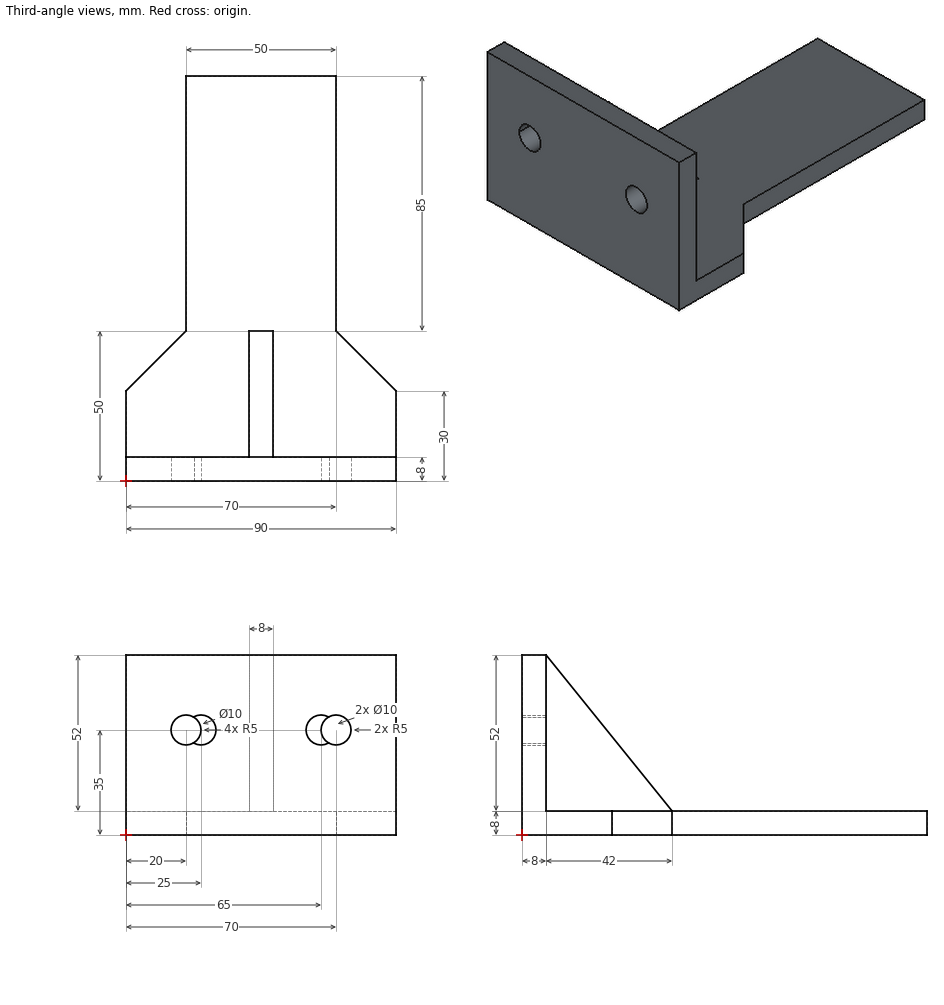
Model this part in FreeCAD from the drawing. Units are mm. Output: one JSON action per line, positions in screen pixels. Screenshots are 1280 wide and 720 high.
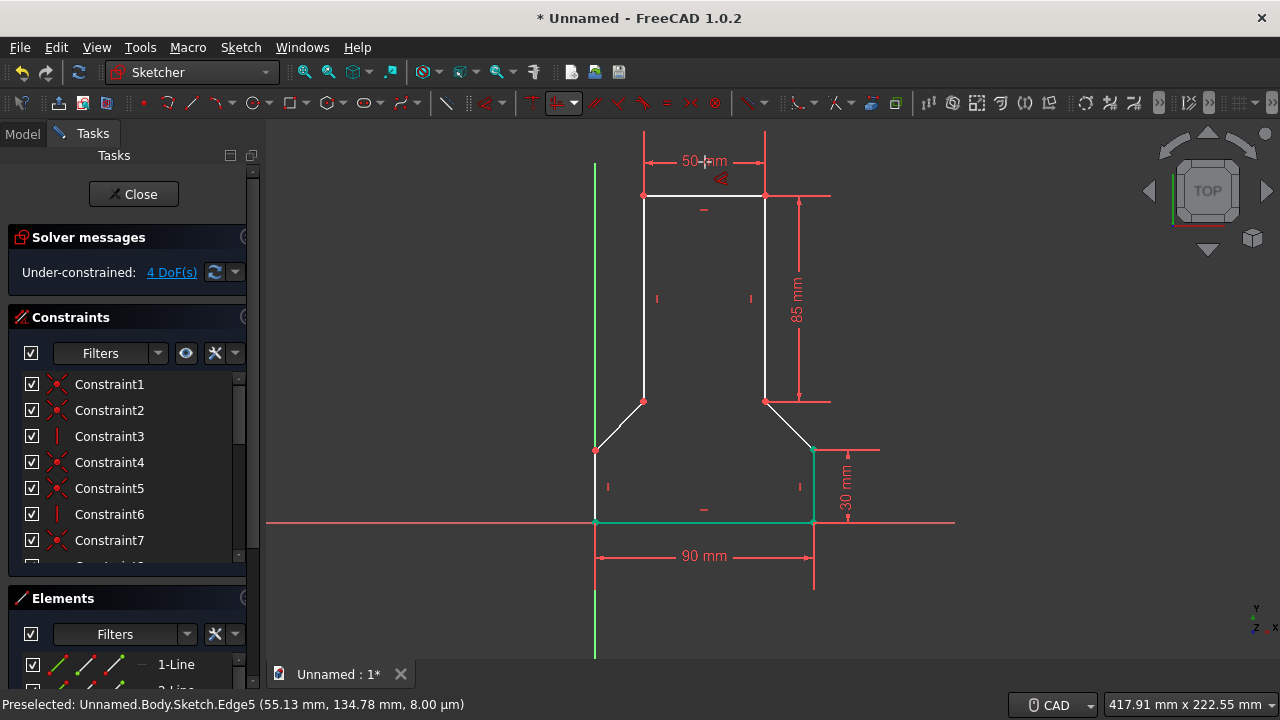
{"action": "left_click", "coordinate": [644, 258]}
{"action": "left_click", "coordinate": [610, 299]}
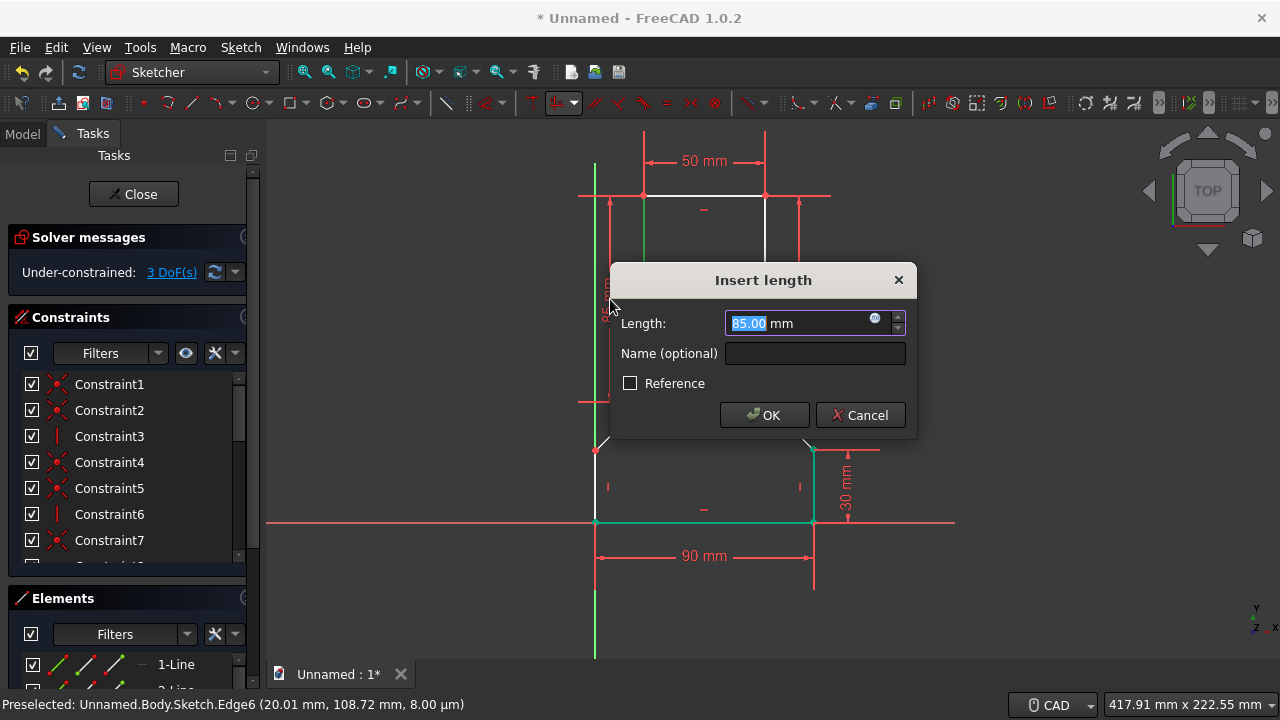
{"action": "type", "text": "85"}
{"action": "key", "text": "Return"}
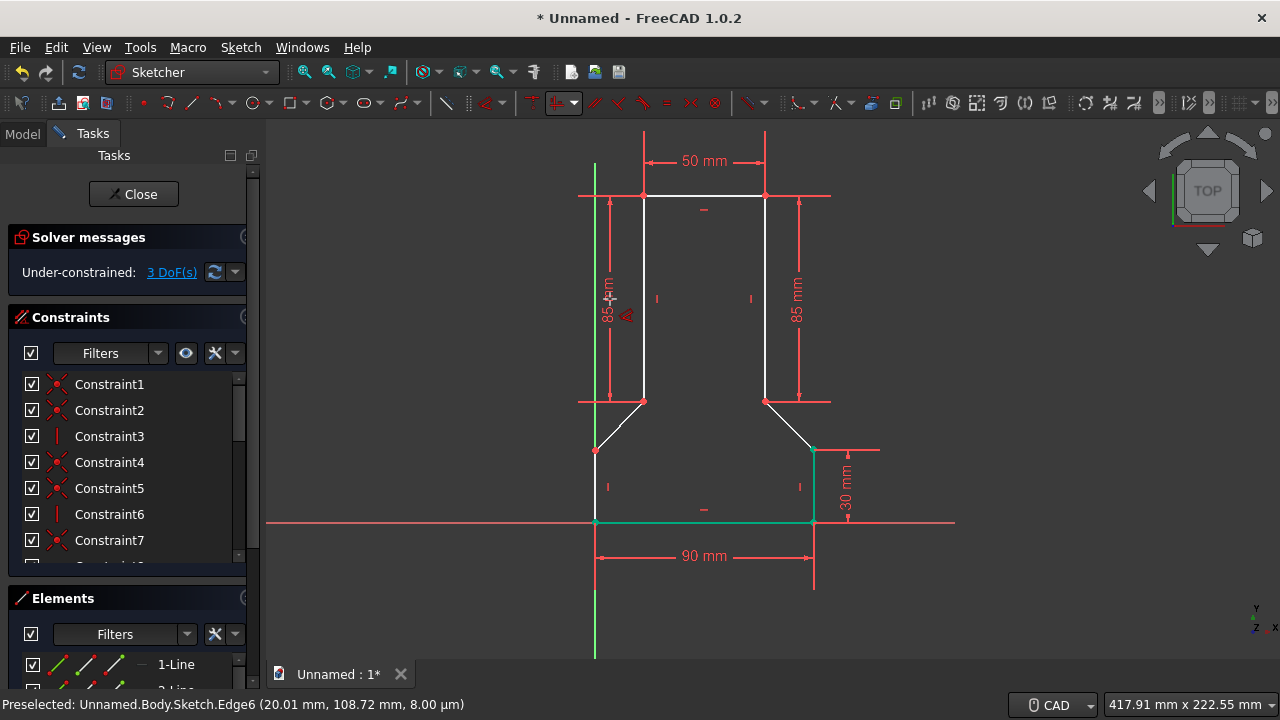
{"action": "left_click", "coordinate": [595, 473]}
{"action": "left_click", "coordinate": [561, 487]}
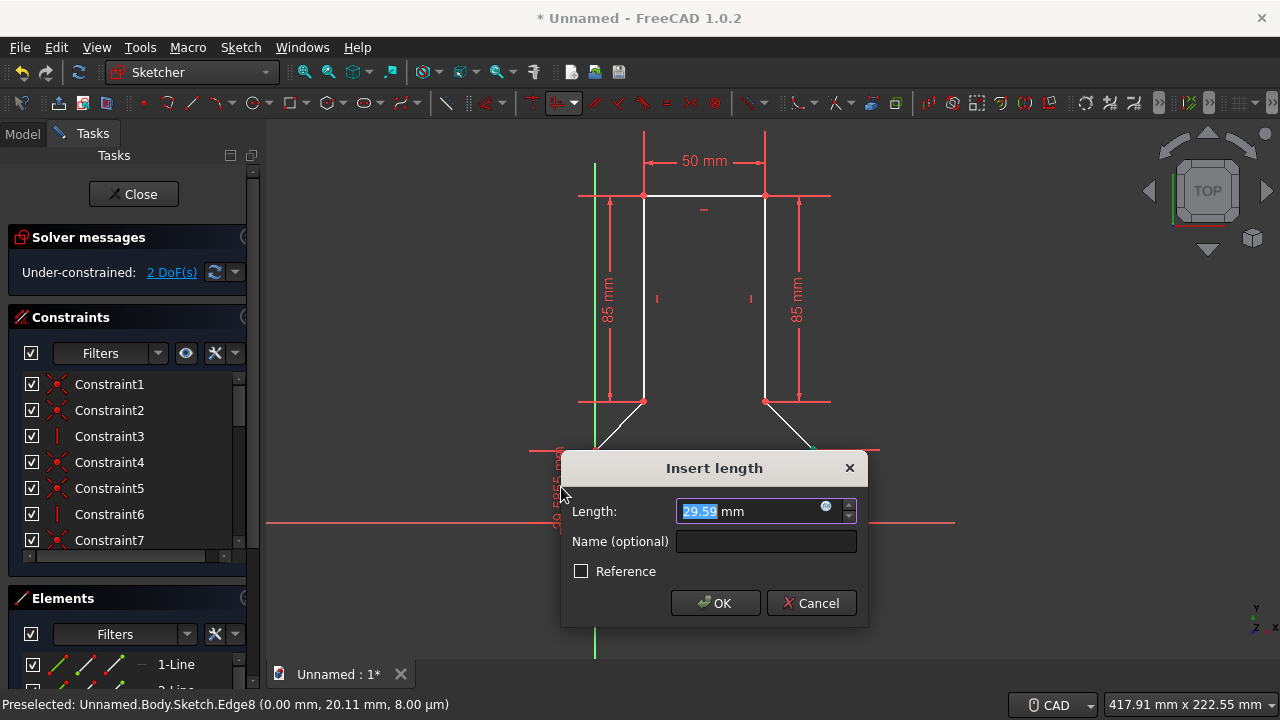
{"action": "type", "text": "30"}
{"action": "key", "text": "Return"}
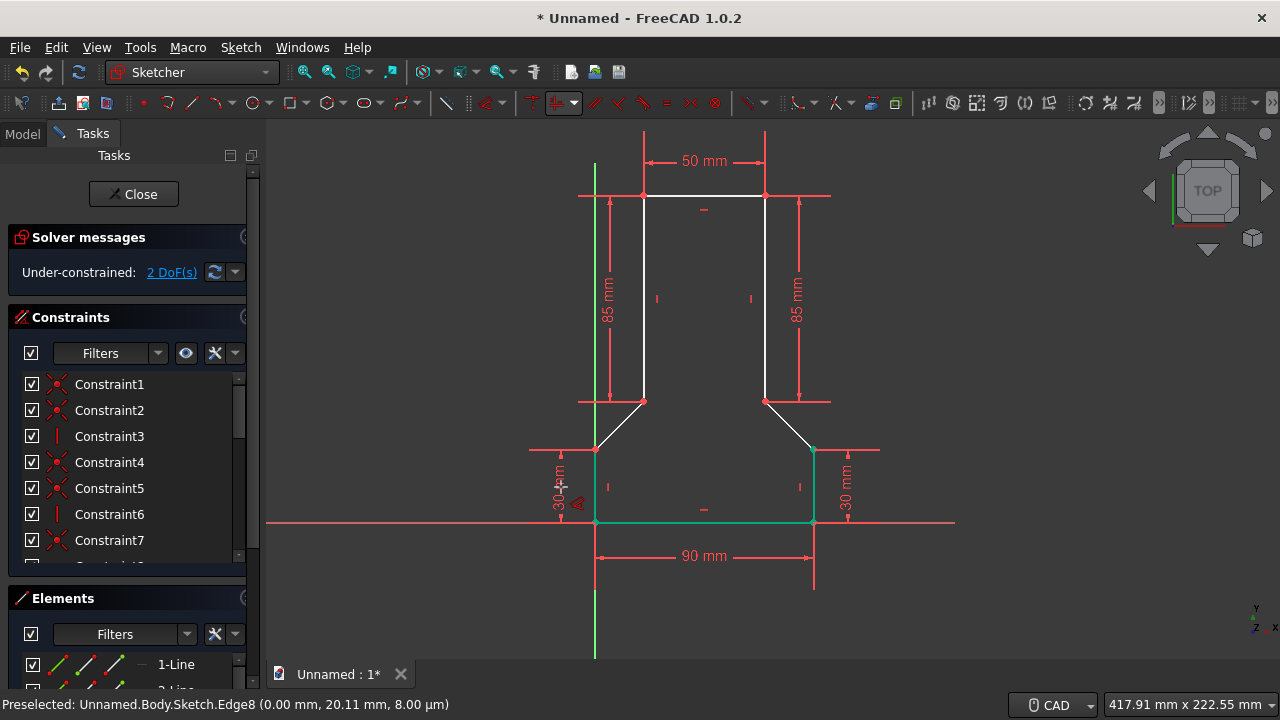
{"action": "left_click", "coordinate": [765, 402]}
{"action": "left_click", "coordinate": [621, 557]}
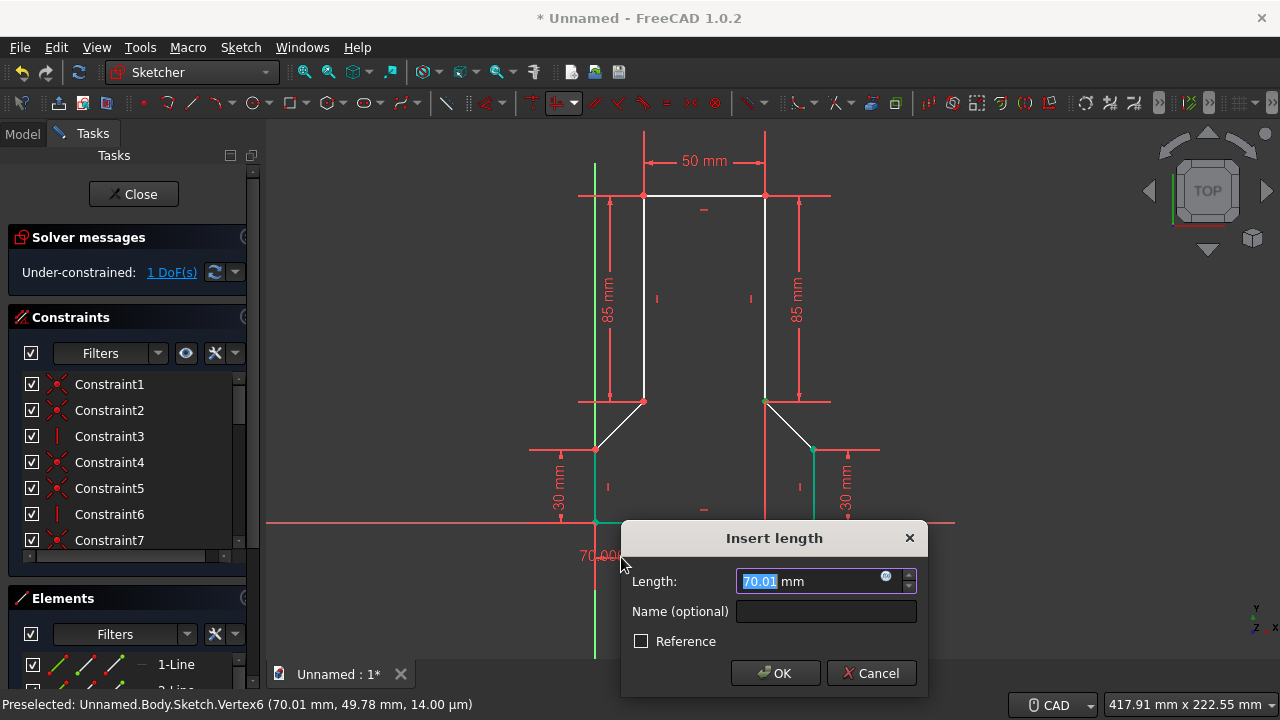
{"action": "type", "text": "70"}
{"action": "key", "text": "Return"}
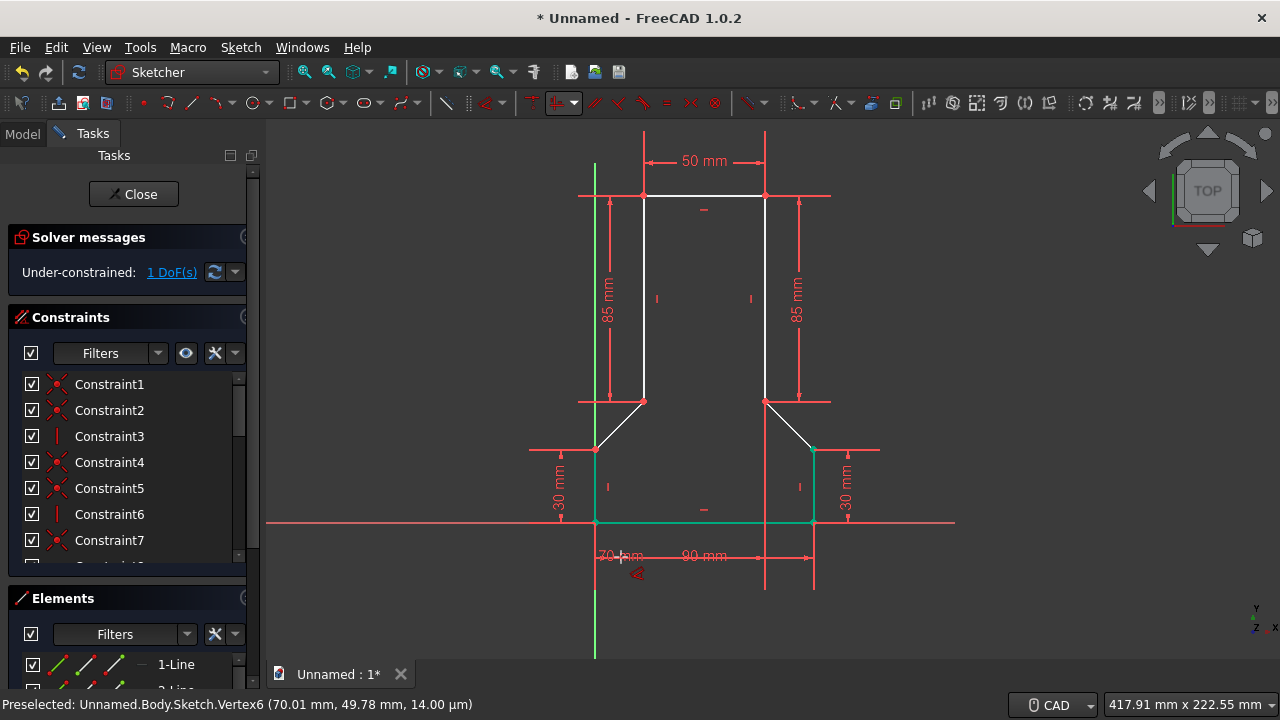
{"action": "left_click", "coordinate": [765, 402]}
{"action": "left_click", "coordinate": [561, 462]}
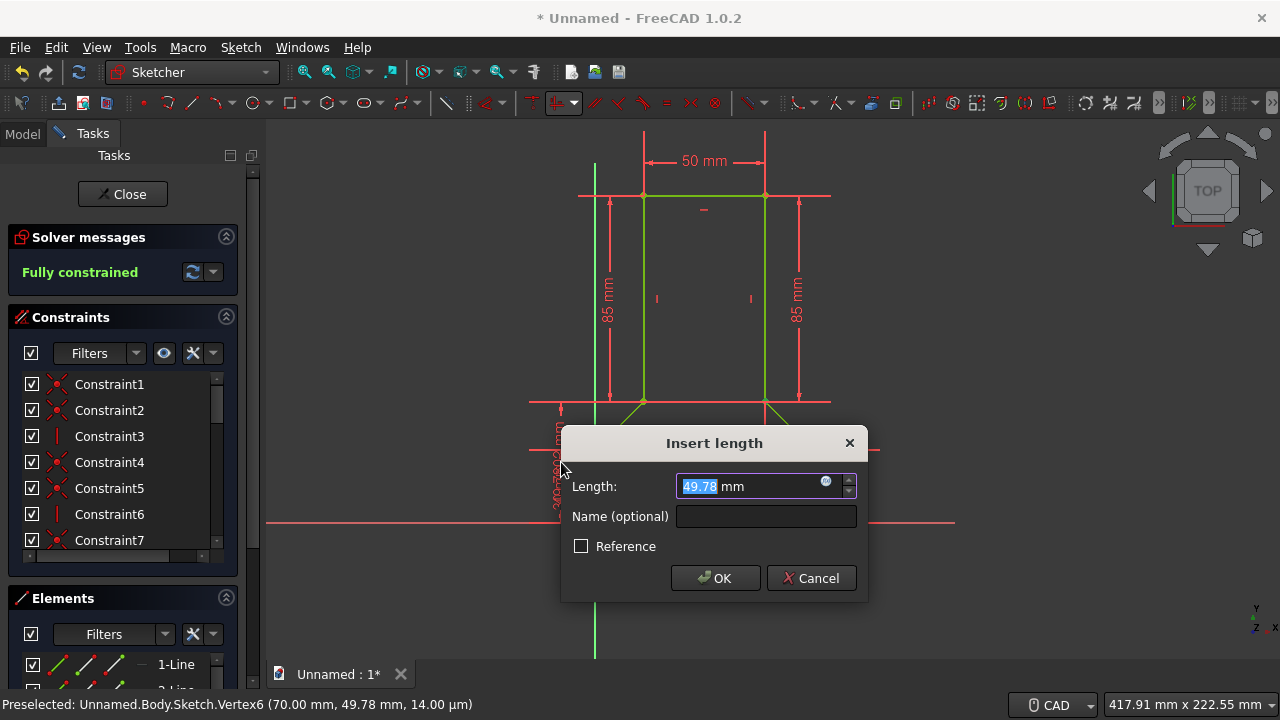
{"action": "type", "text": "50"}
{"action": "key", "text": "Return"}
{"action": "key", "text": "Escape"}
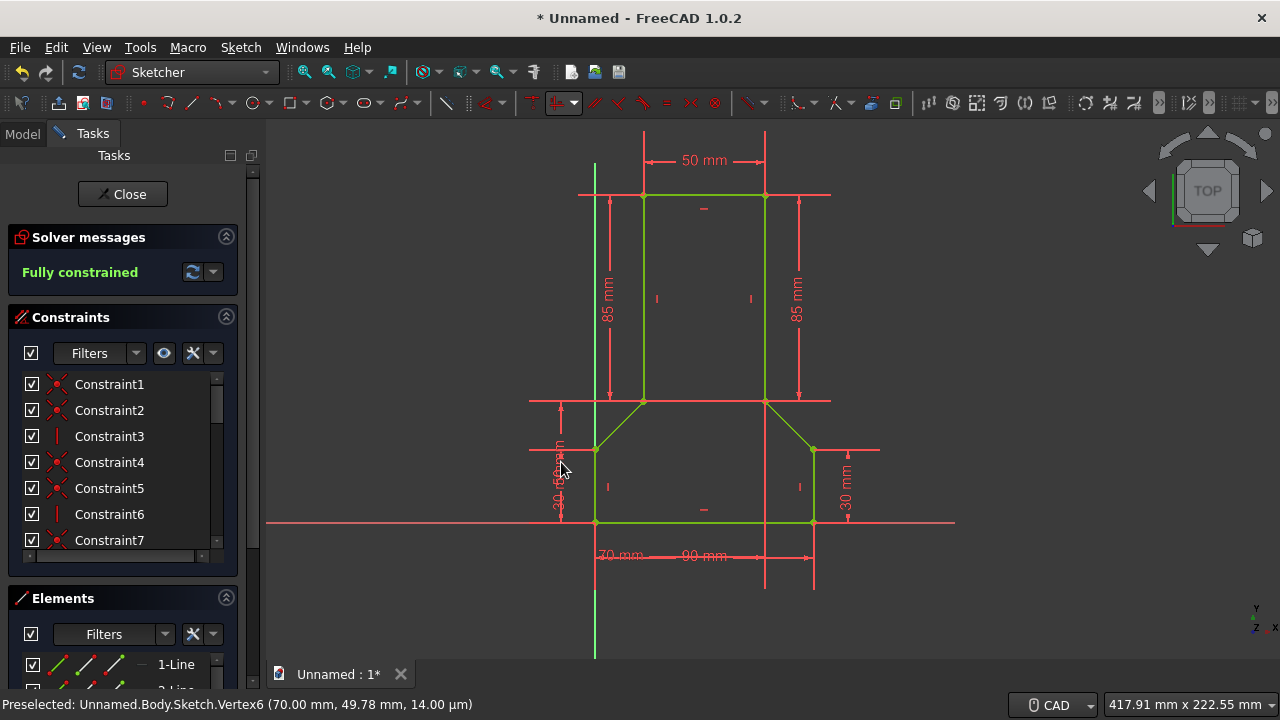
{"action": "left_click", "coordinate": [123, 194]}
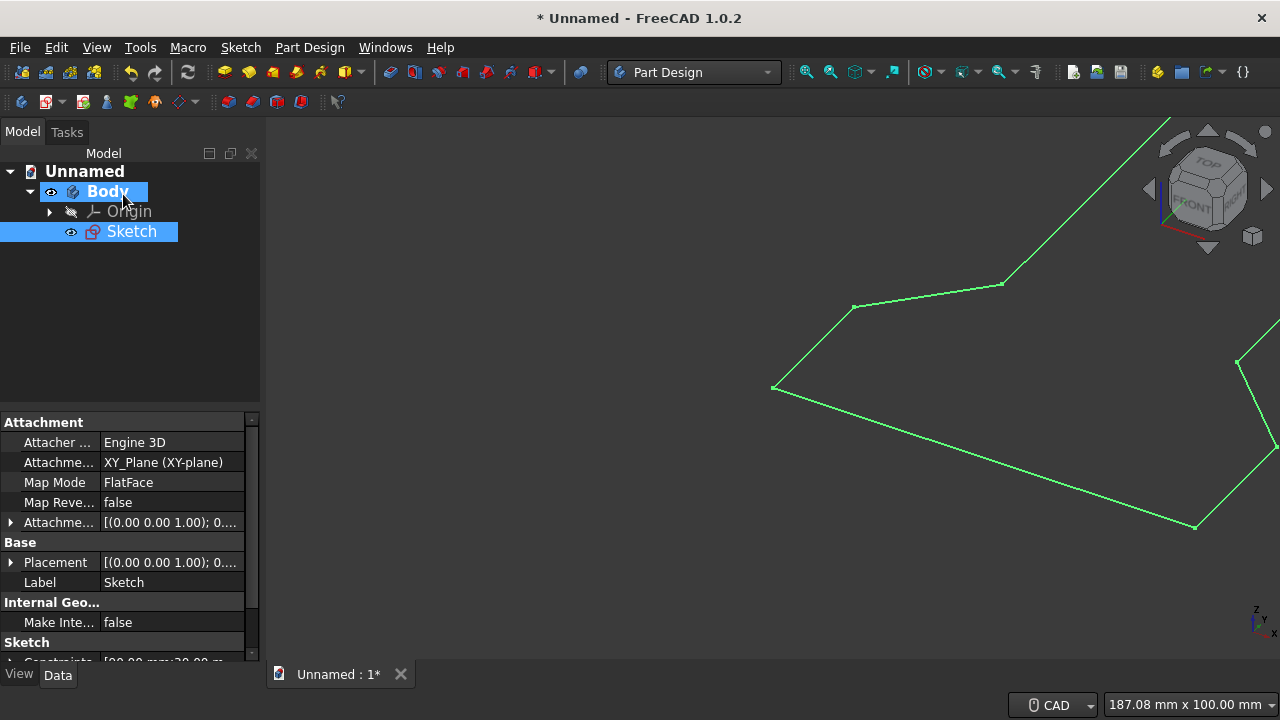
{"action": "left_click", "coordinate": [226, 72]}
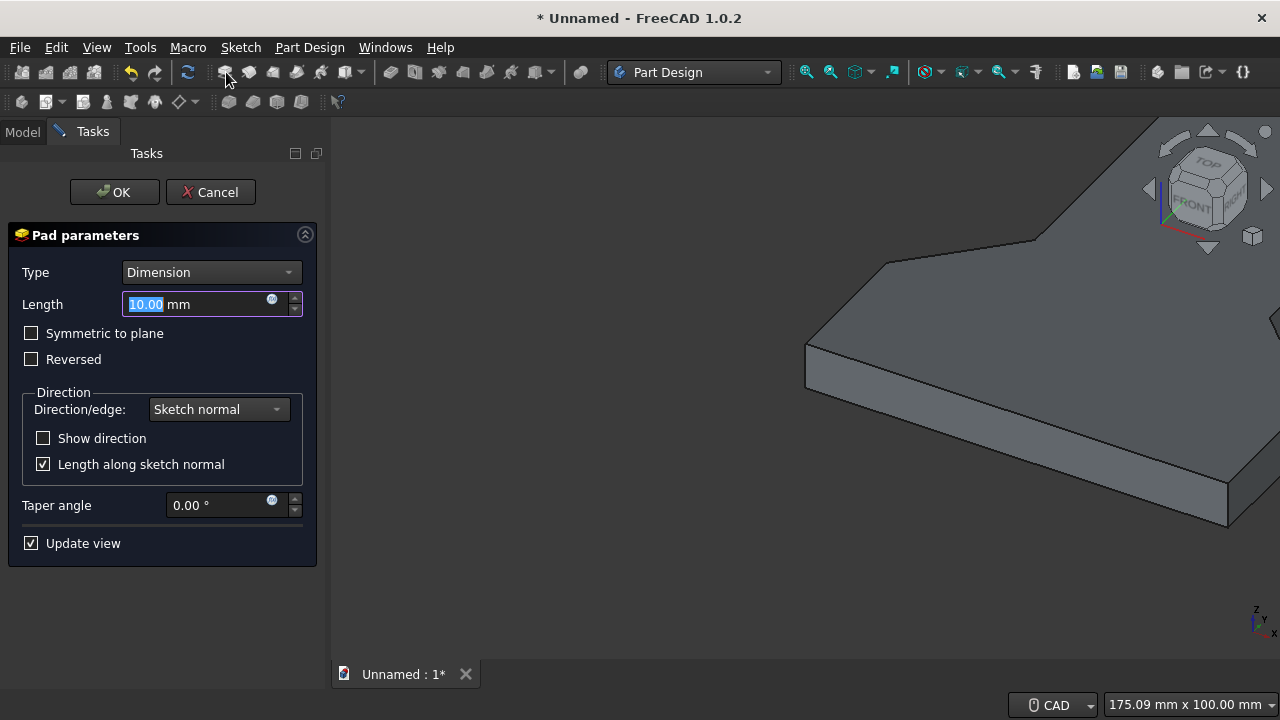
{"action": "type", "text": "8"}
{"action": "key", "text": "Tab"}